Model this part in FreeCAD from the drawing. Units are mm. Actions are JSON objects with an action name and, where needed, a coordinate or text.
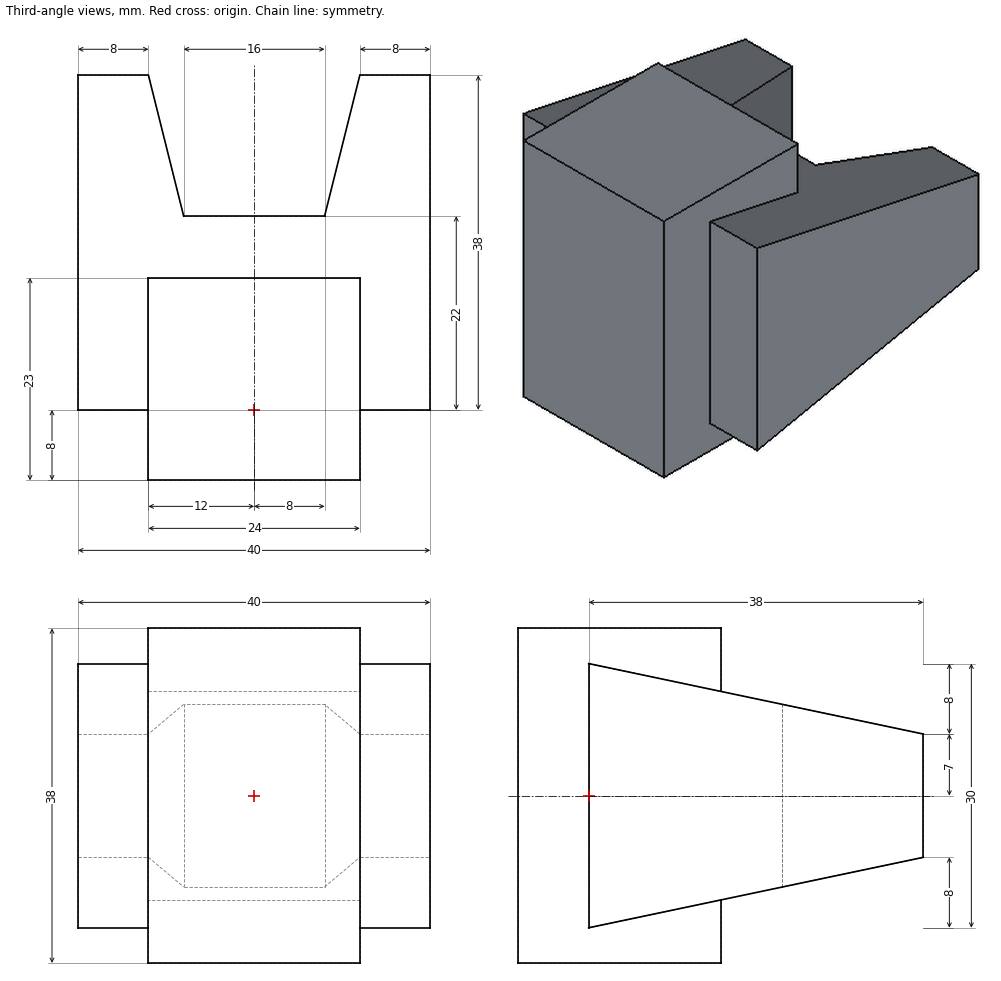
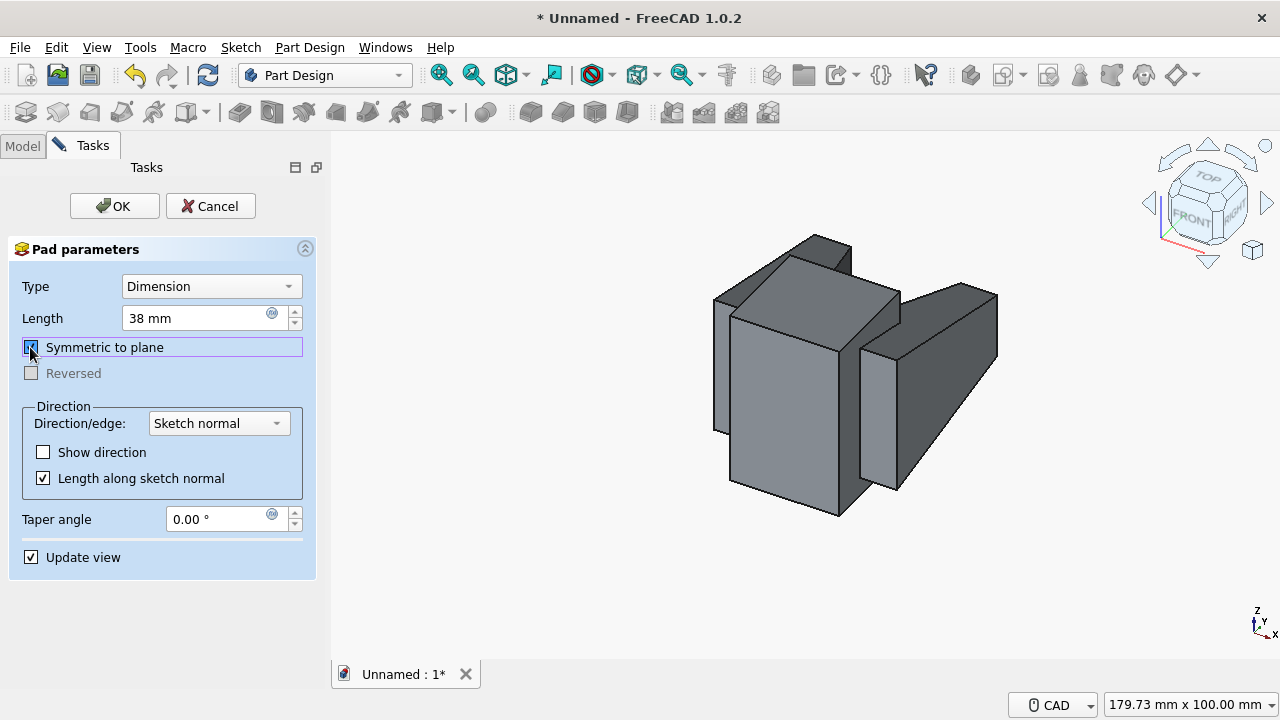
{"action": "left_click", "coordinate": [115, 206]}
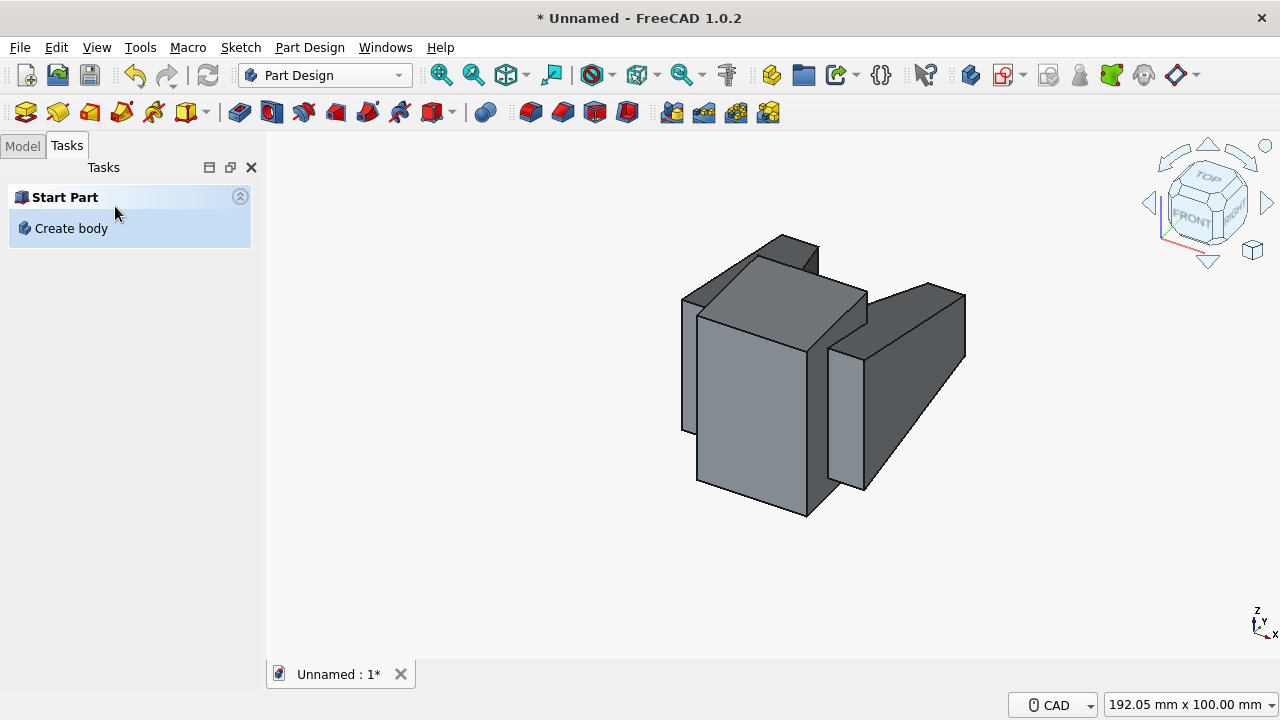
{"action": "key", "text": "0"}